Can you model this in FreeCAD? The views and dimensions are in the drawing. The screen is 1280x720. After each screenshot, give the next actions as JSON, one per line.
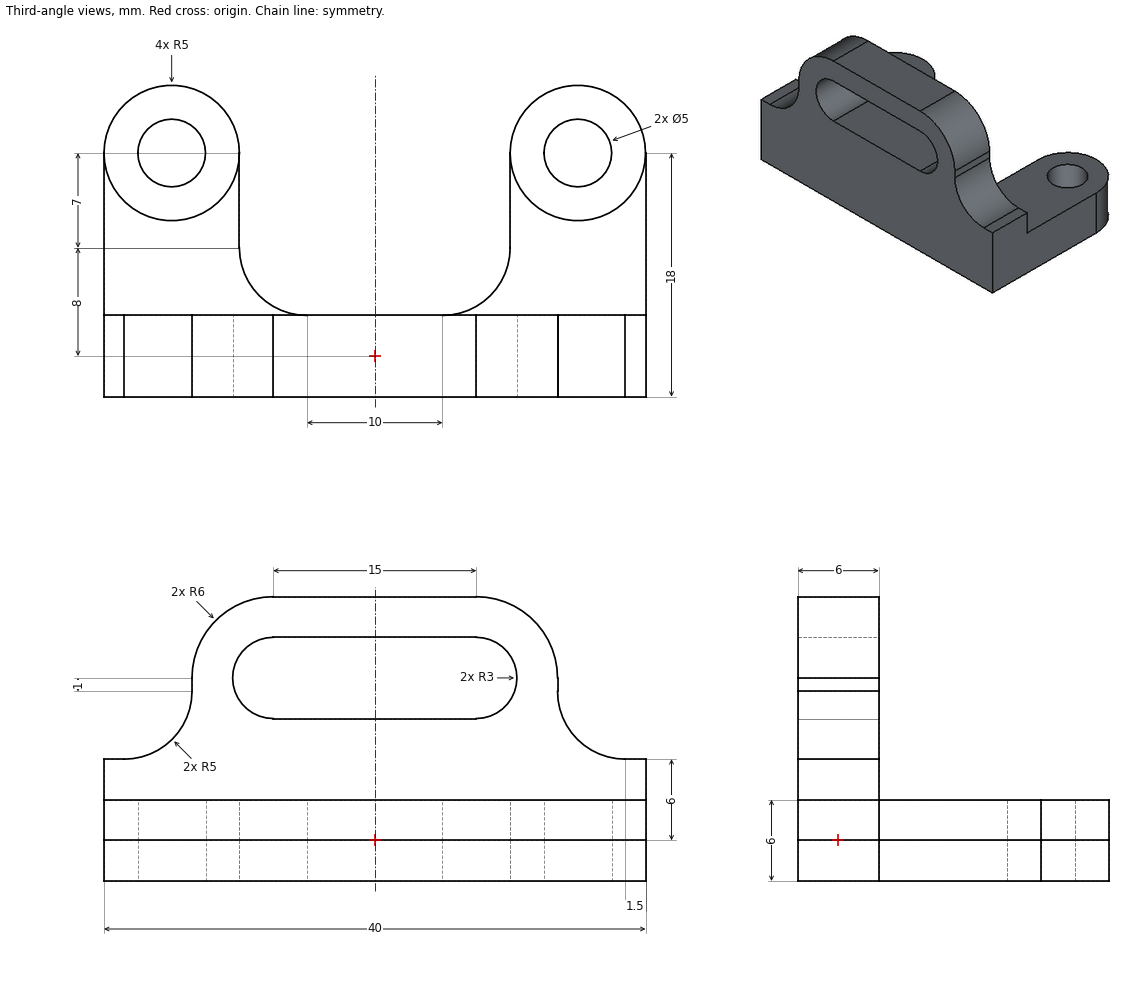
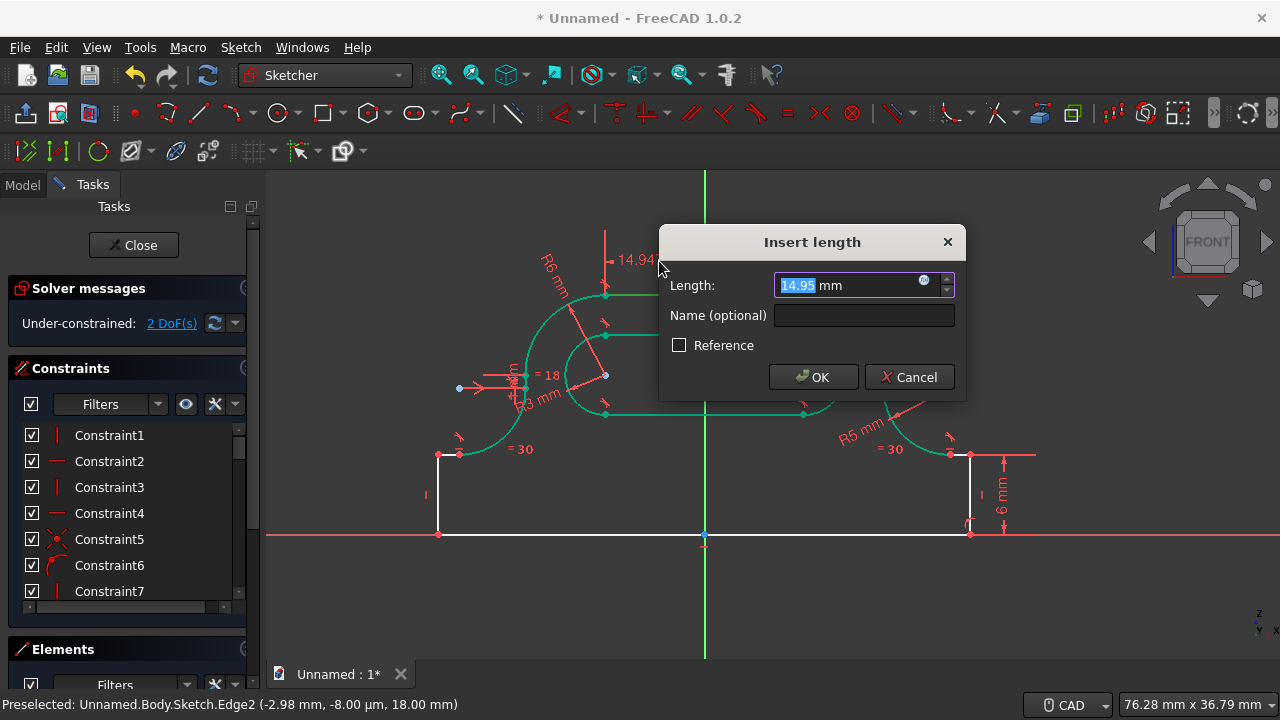
{"action": "type", "text": "15"}
{"action": "key", "text": "Return"}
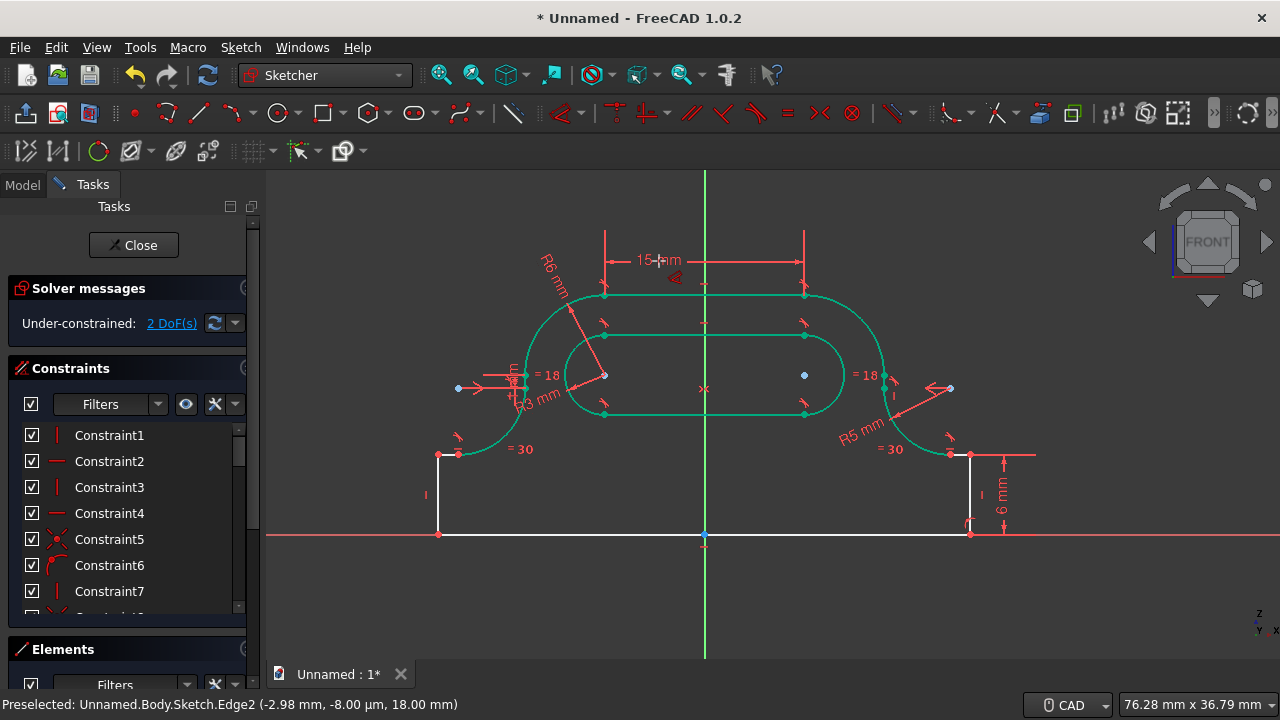
{"action": "left_click", "coordinate": [811, 535]}
{"action": "left_click", "coordinate": [582, 569]}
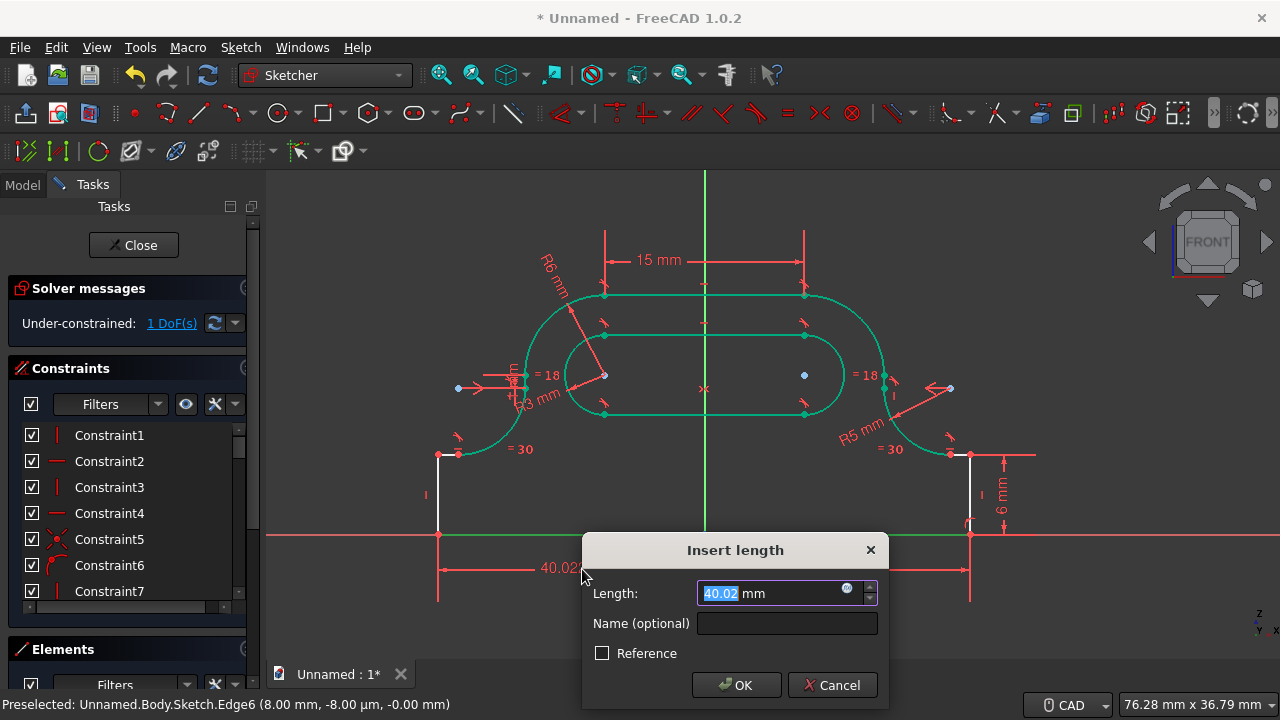
{"action": "type", "text": "40"}
{"action": "key", "text": "Return"}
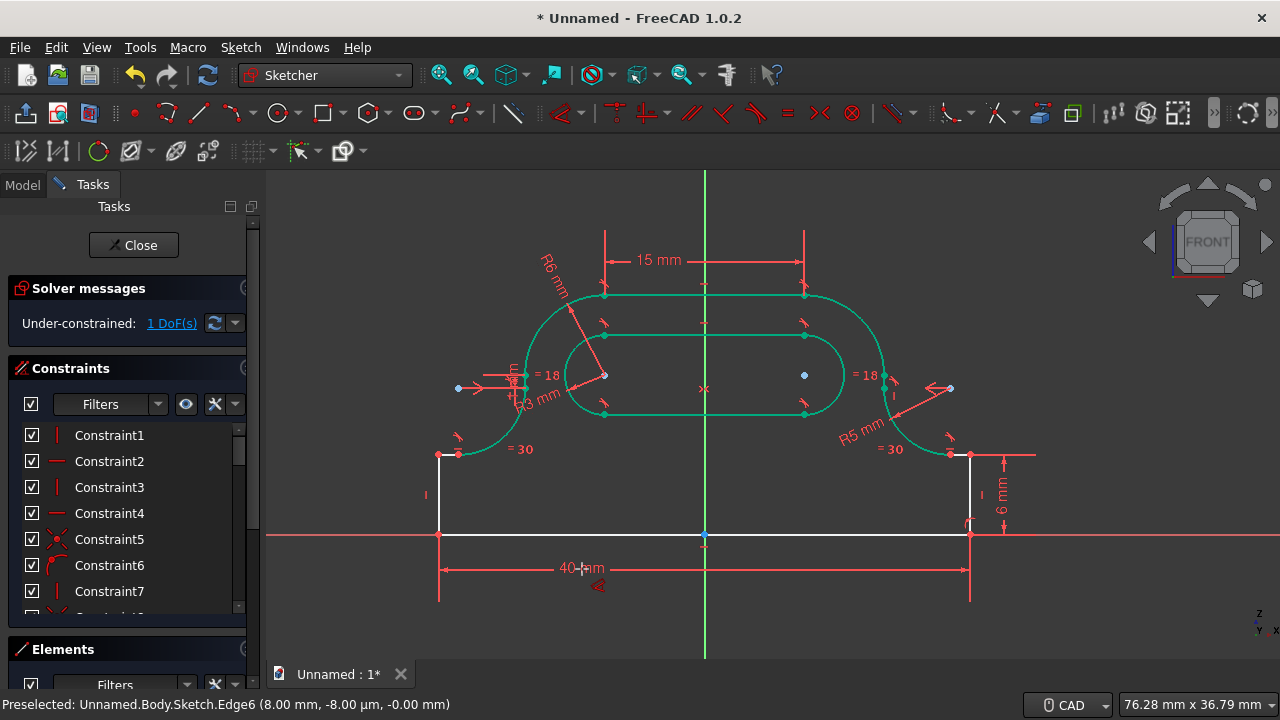
{"action": "scroll", "coordinate": [960, 455], "scroll_direction": "up", "scroll_amount": 4}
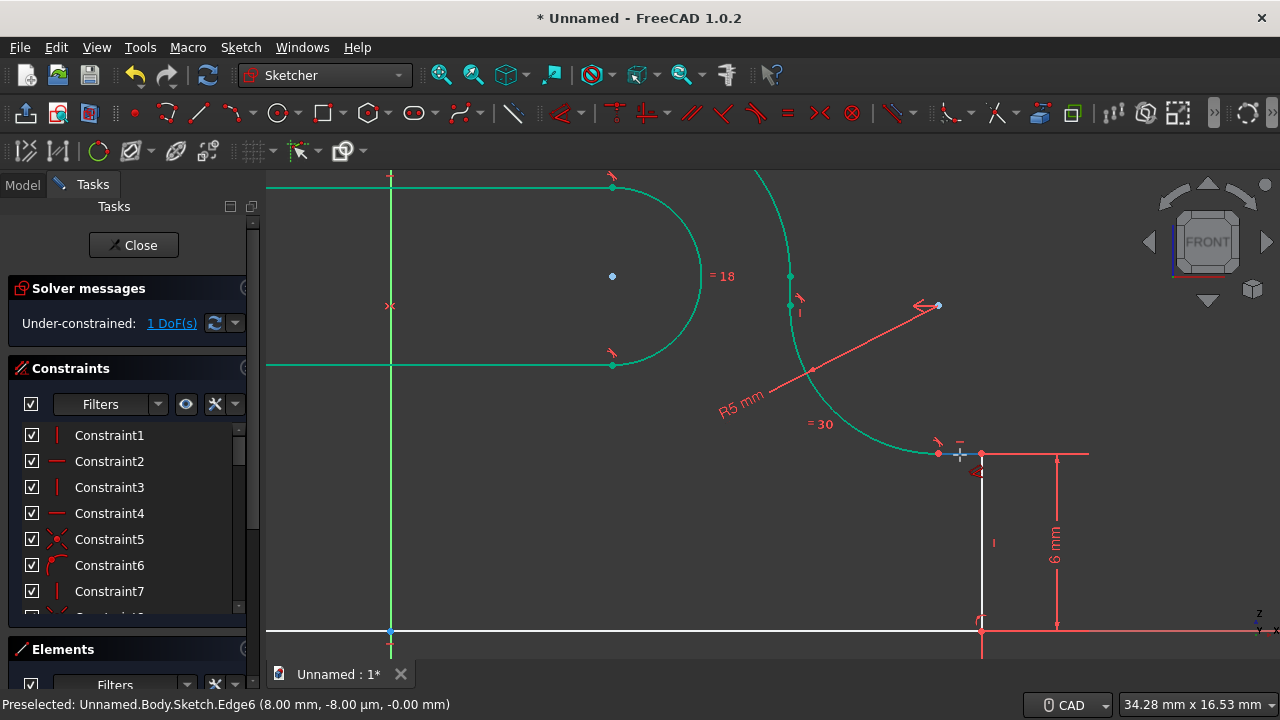
{"action": "left_click", "coordinate": [960, 454]}
{"action": "left_click", "coordinate": [960, 488]}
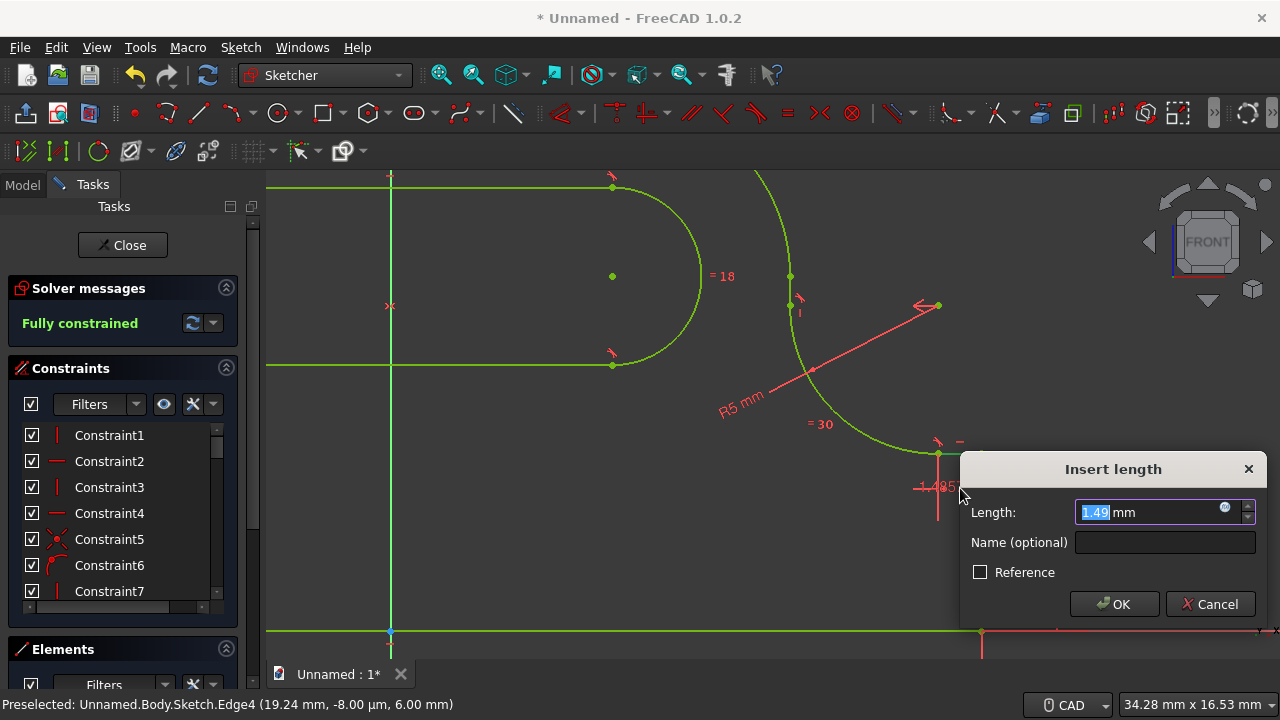
{"action": "type", "text": "1.5"}
{"action": "key", "text": "Return"}
{"action": "key", "text": "Escape"}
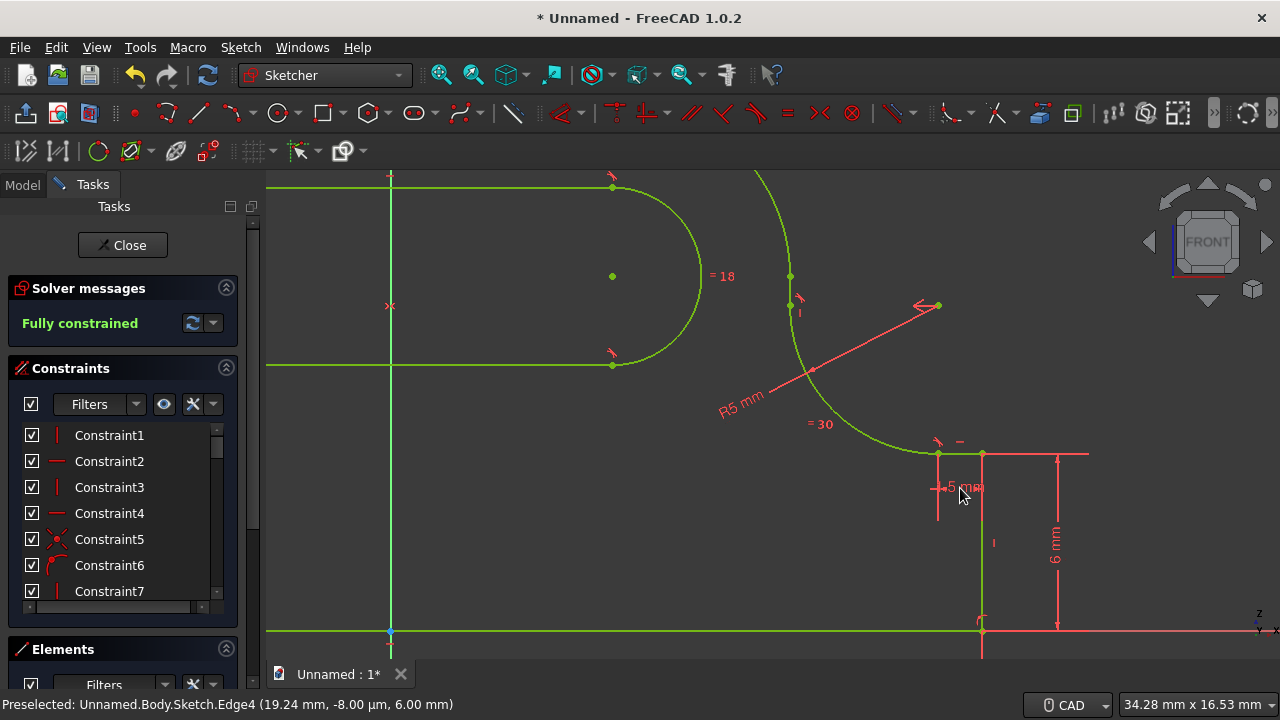
{"action": "left_click", "coordinate": [123, 245]}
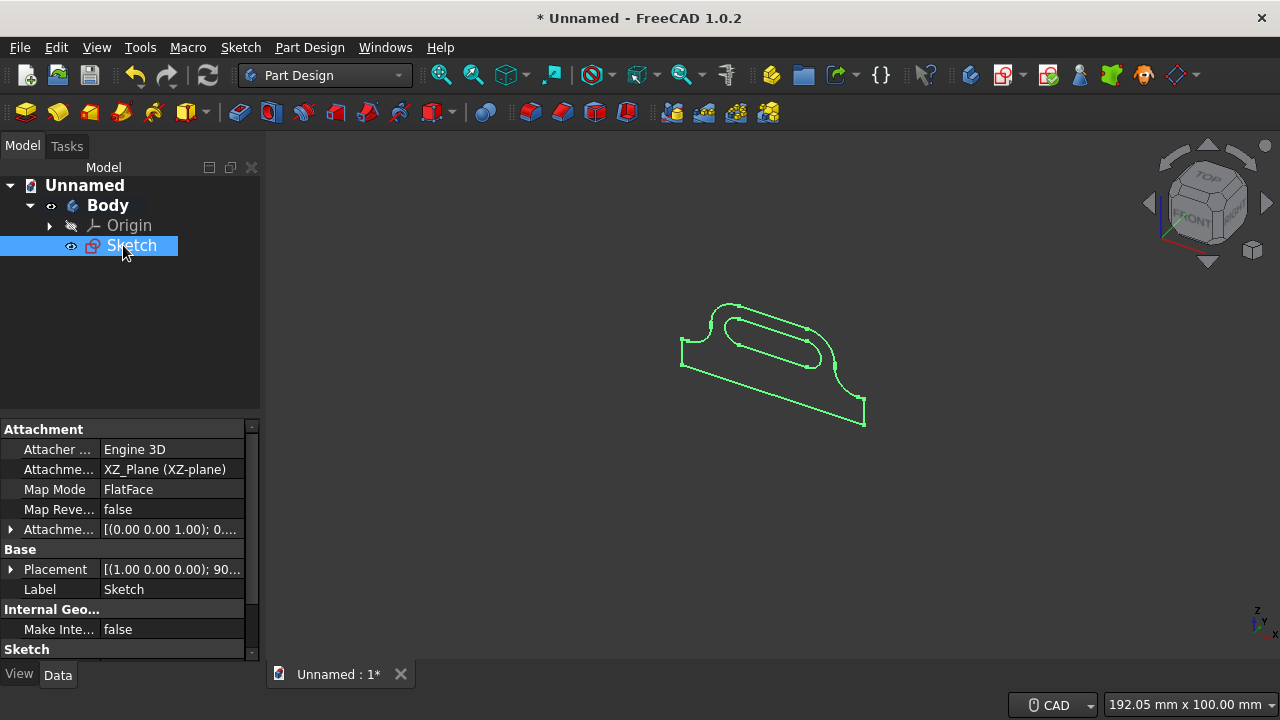
{"action": "left_click", "coordinate": [26, 112]}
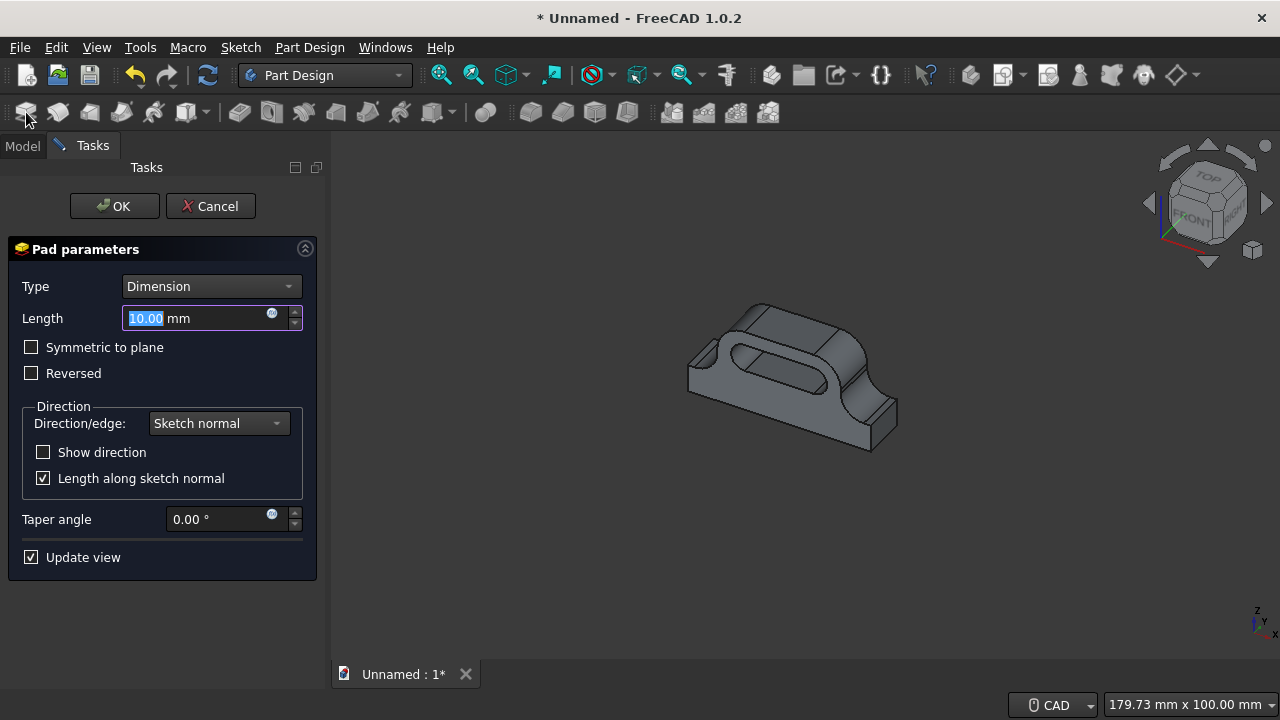
{"action": "type", "text": "6"}
{"action": "key", "text": "Tab"}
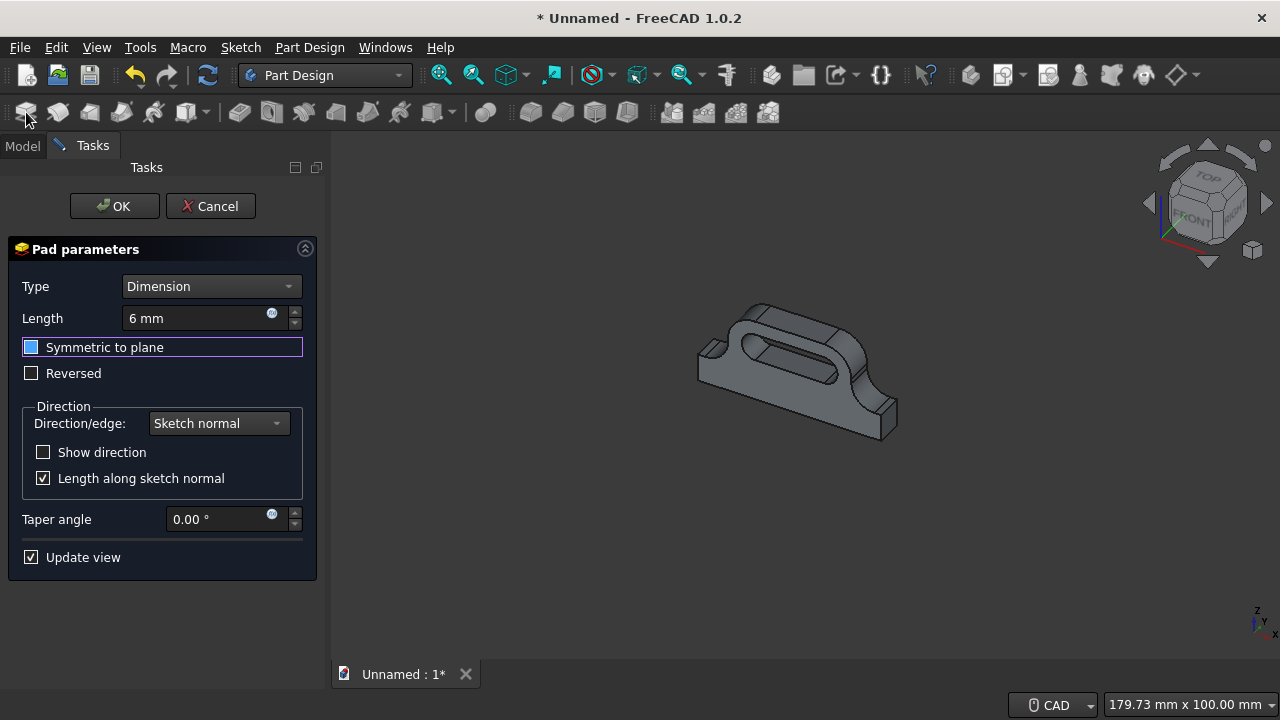
{"action": "left_click", "coordinate": [30, 347]}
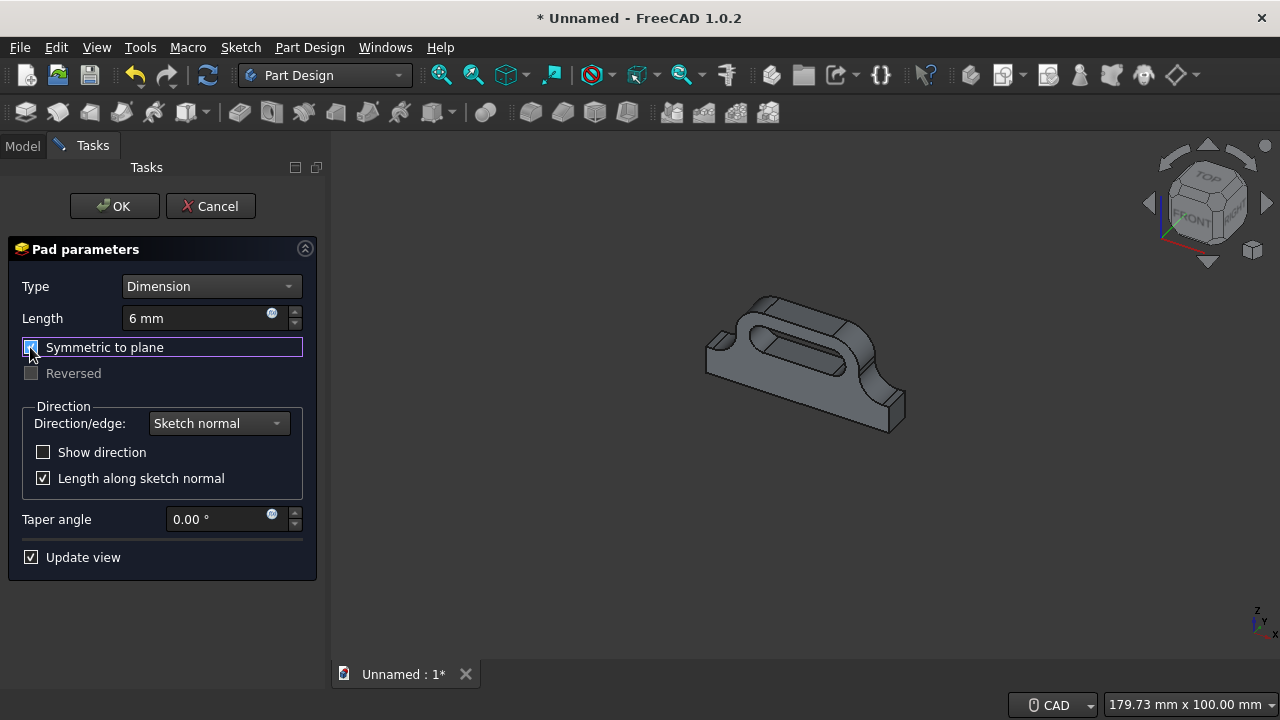
{"action": "left_click", "coordinate": [115, 206]}